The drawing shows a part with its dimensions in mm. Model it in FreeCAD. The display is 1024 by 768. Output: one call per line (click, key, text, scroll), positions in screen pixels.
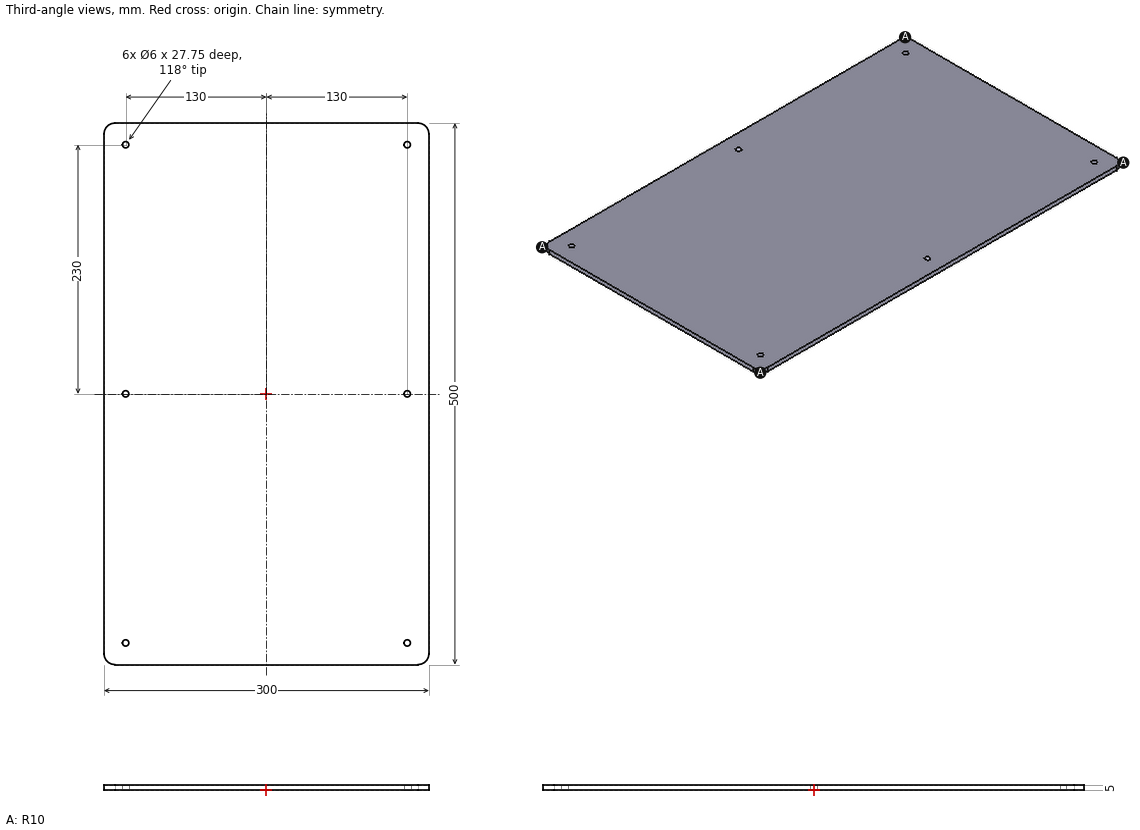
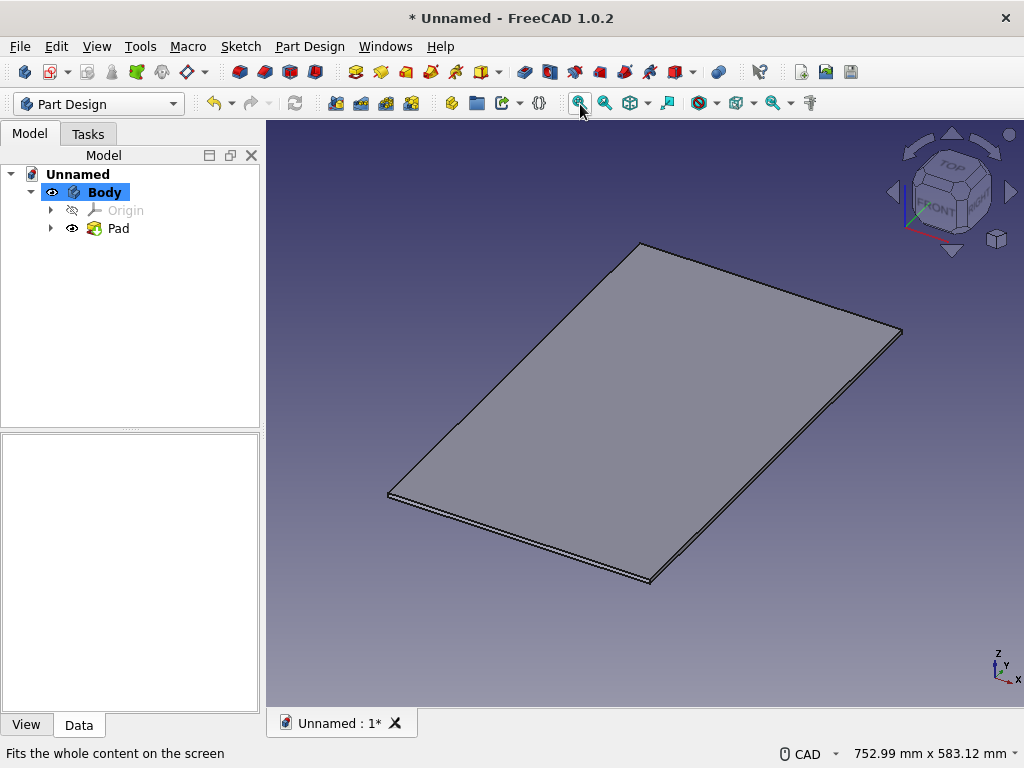
click(681, 375)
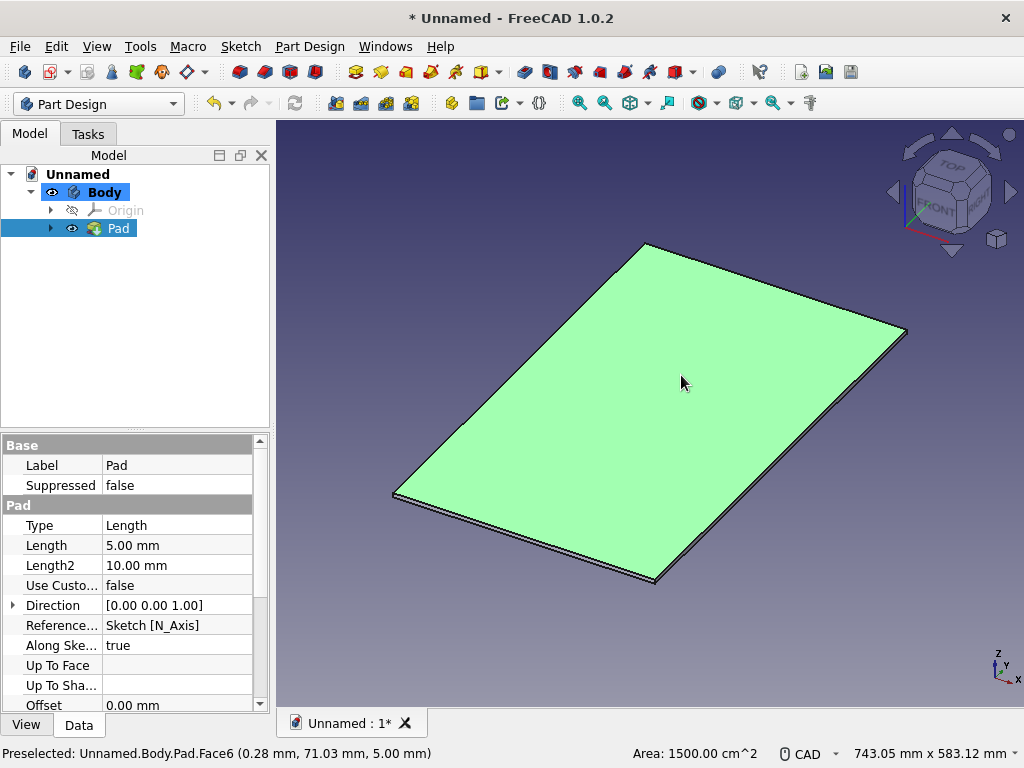
click(50, 72)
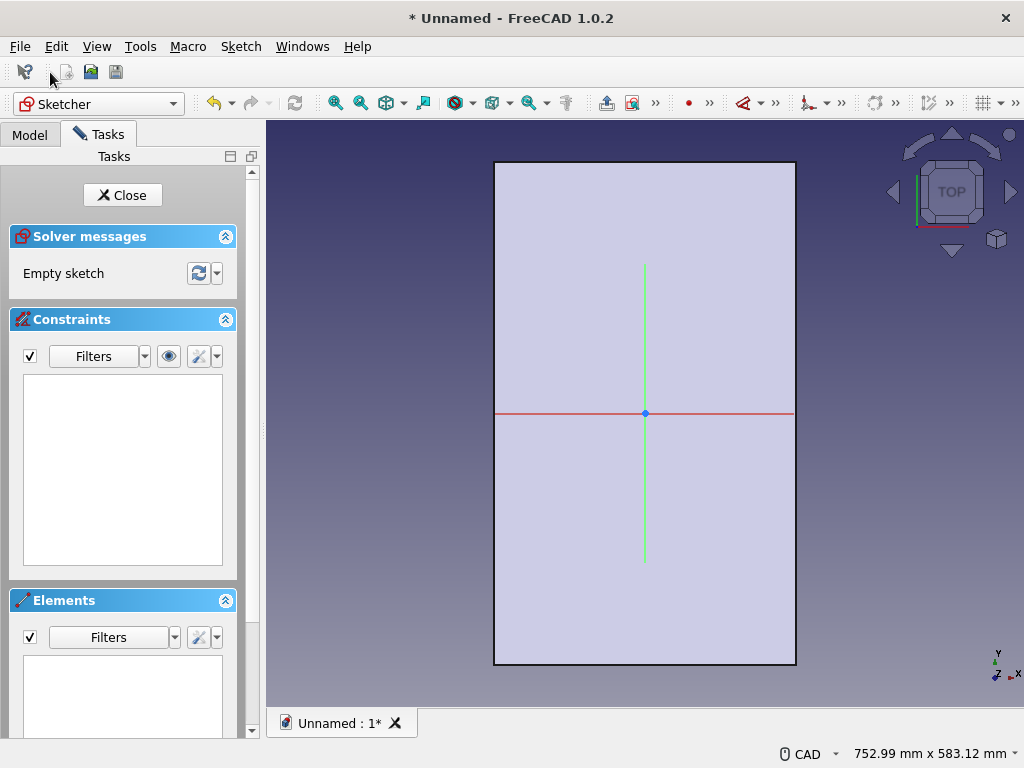
key(g)
key(c)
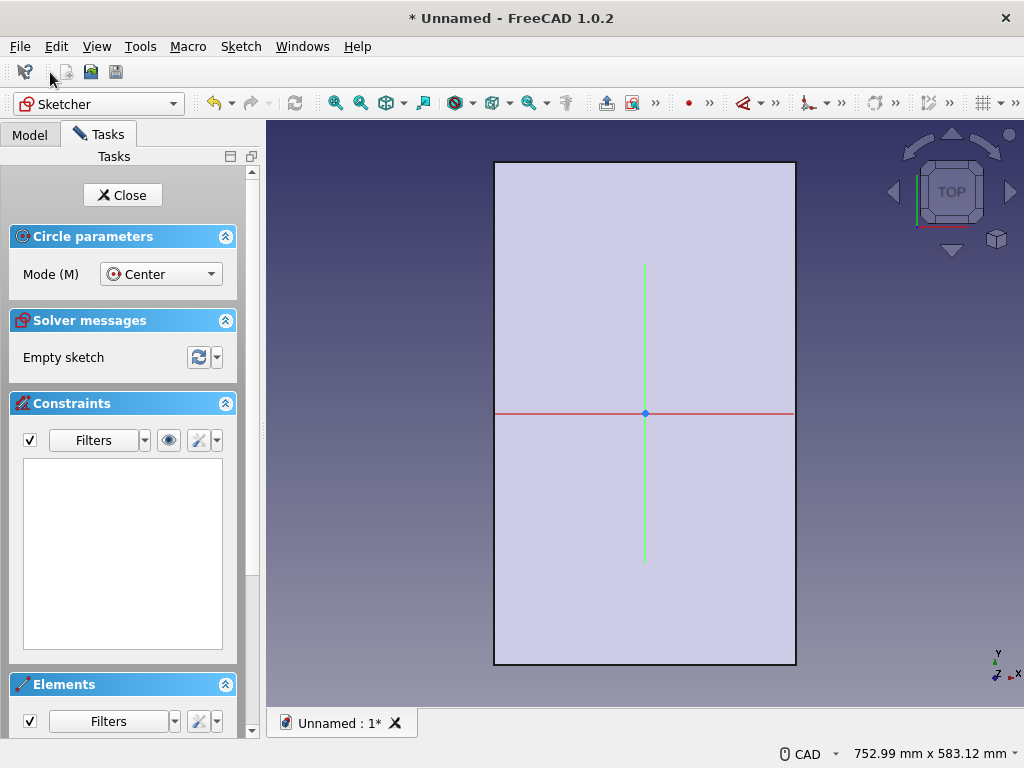
scroll(514, 182, up, 11)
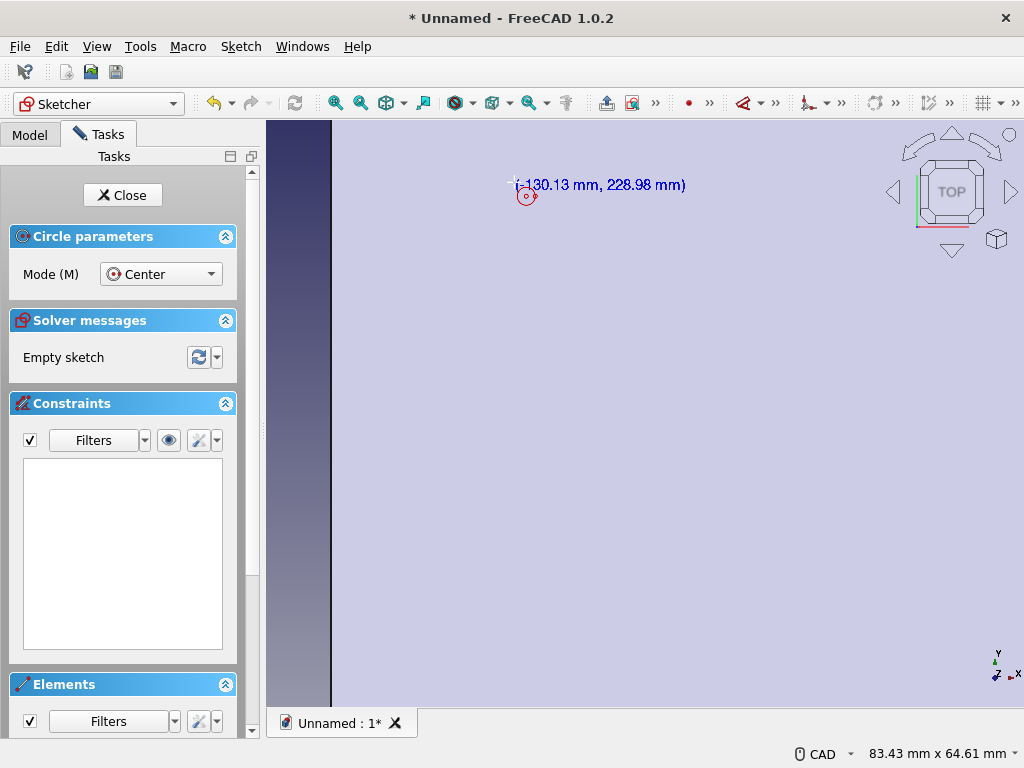
scroll(465, 228, down, 12)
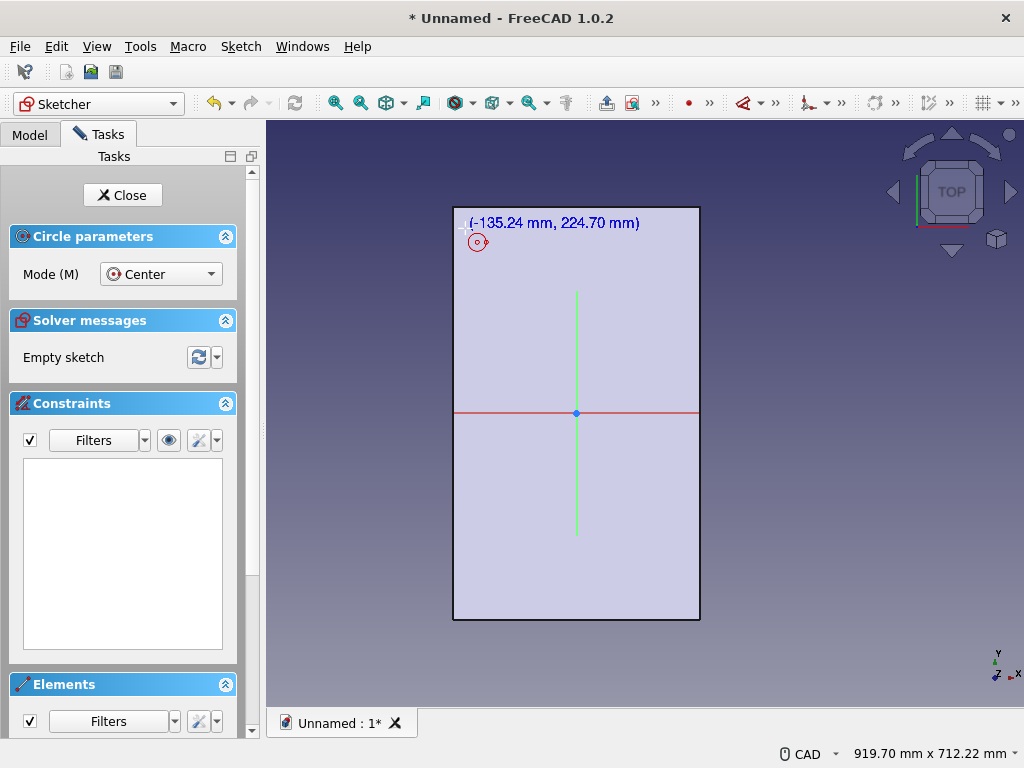
click(470, 224)
move(471, 222)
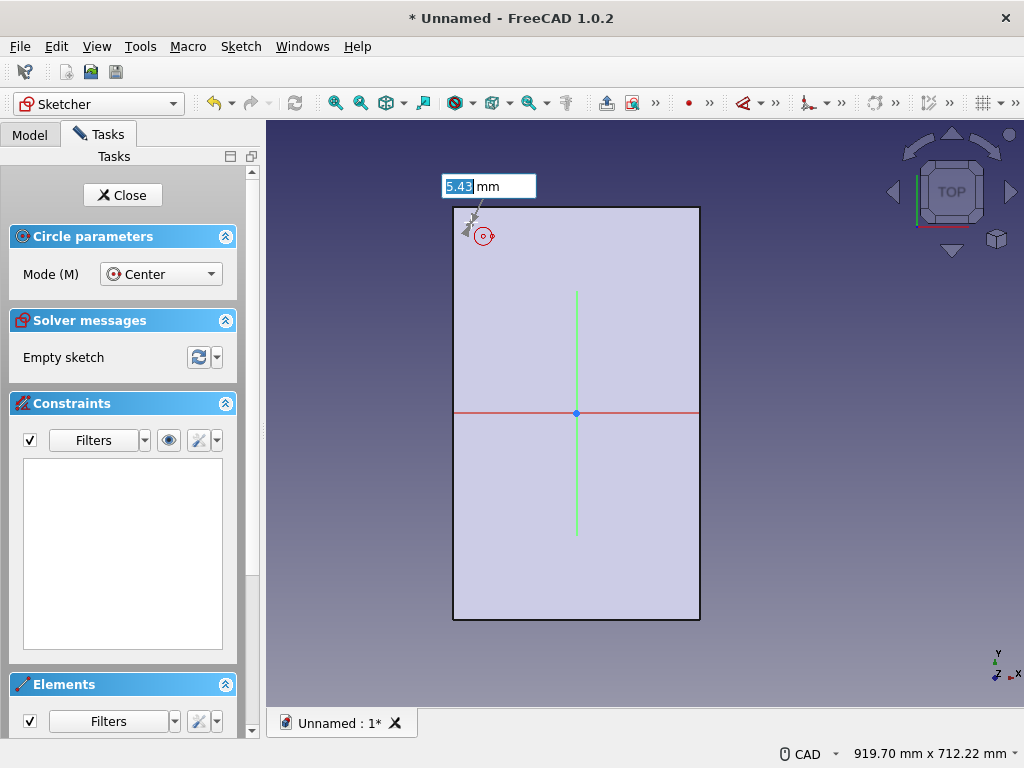
text(6)
key(Return)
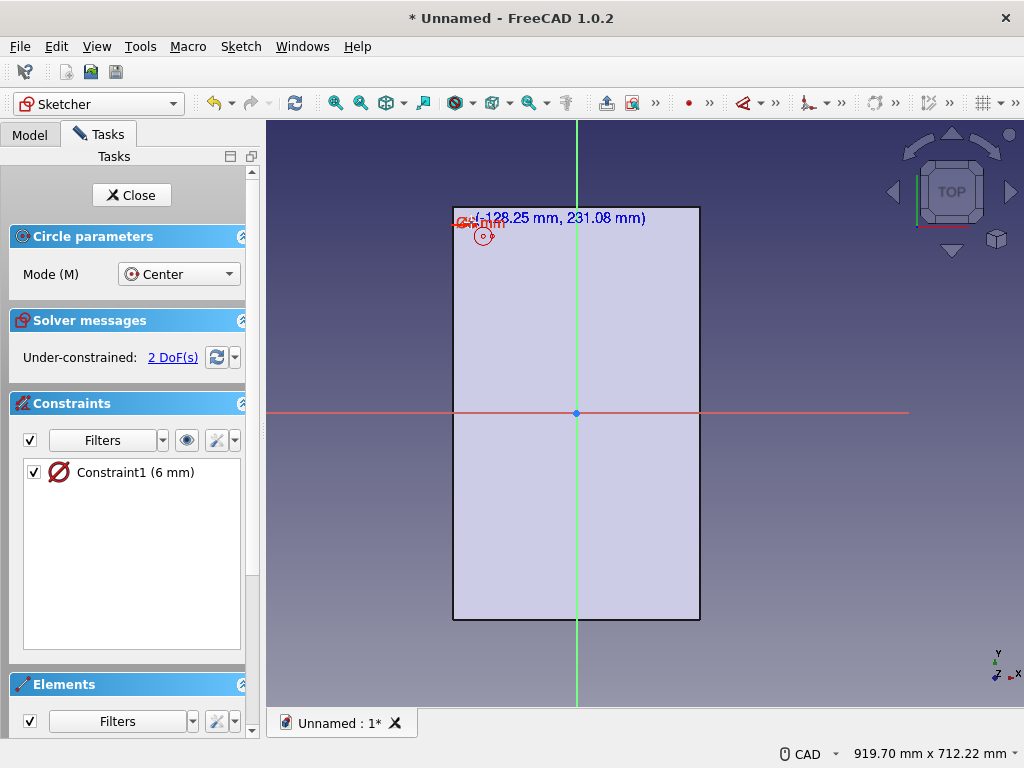
scroll(684, 224, up, 12)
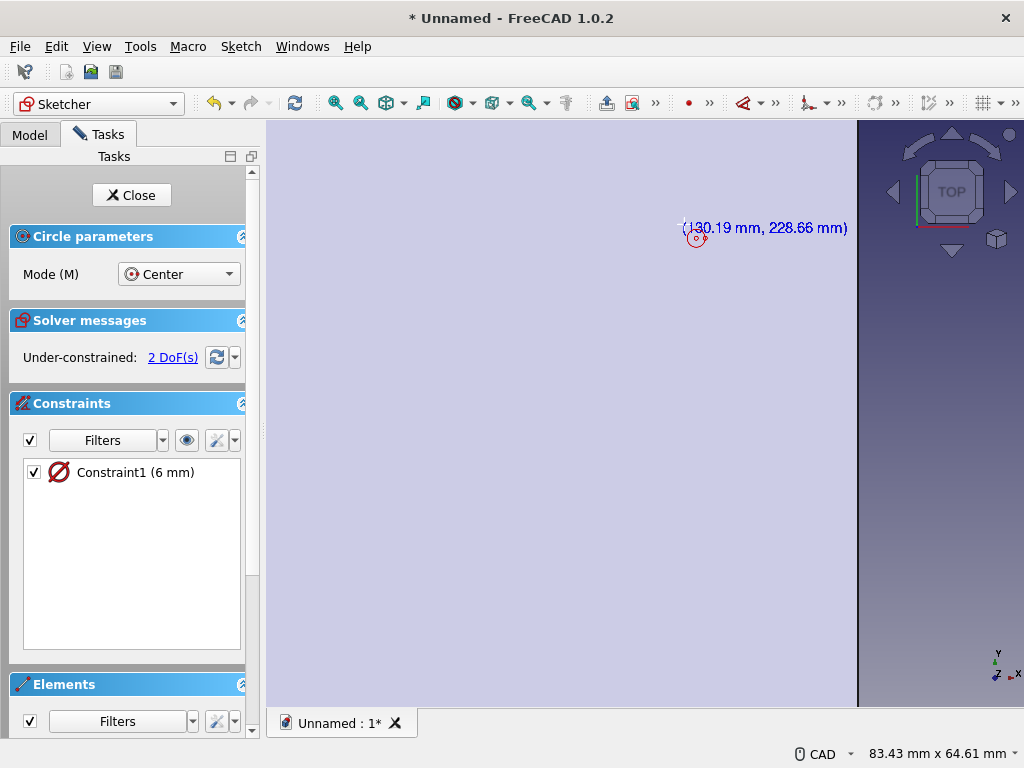
scroll(684, 224, down, 12)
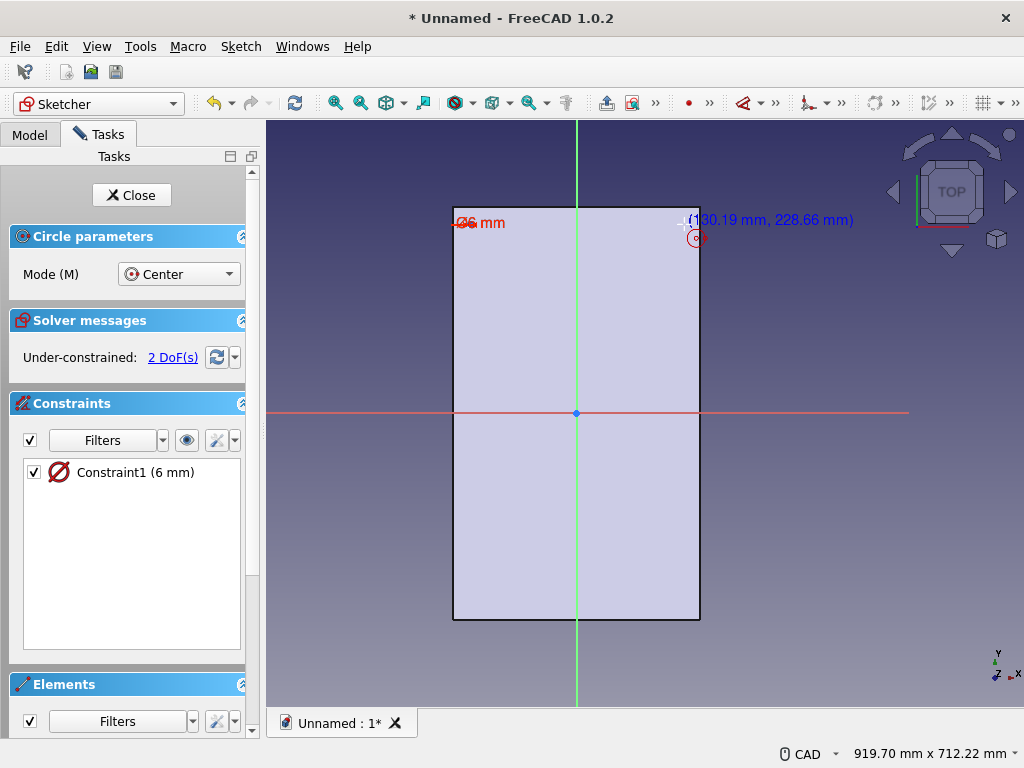
click(684, 224)
move(686, 222)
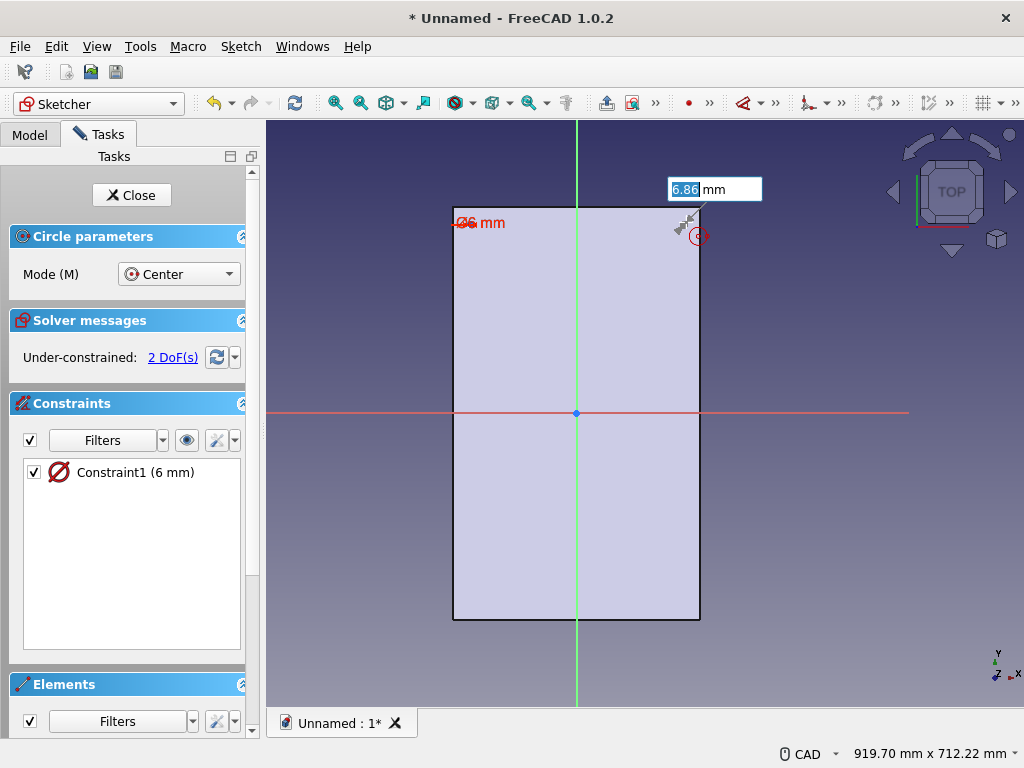
text(6)
key(Return)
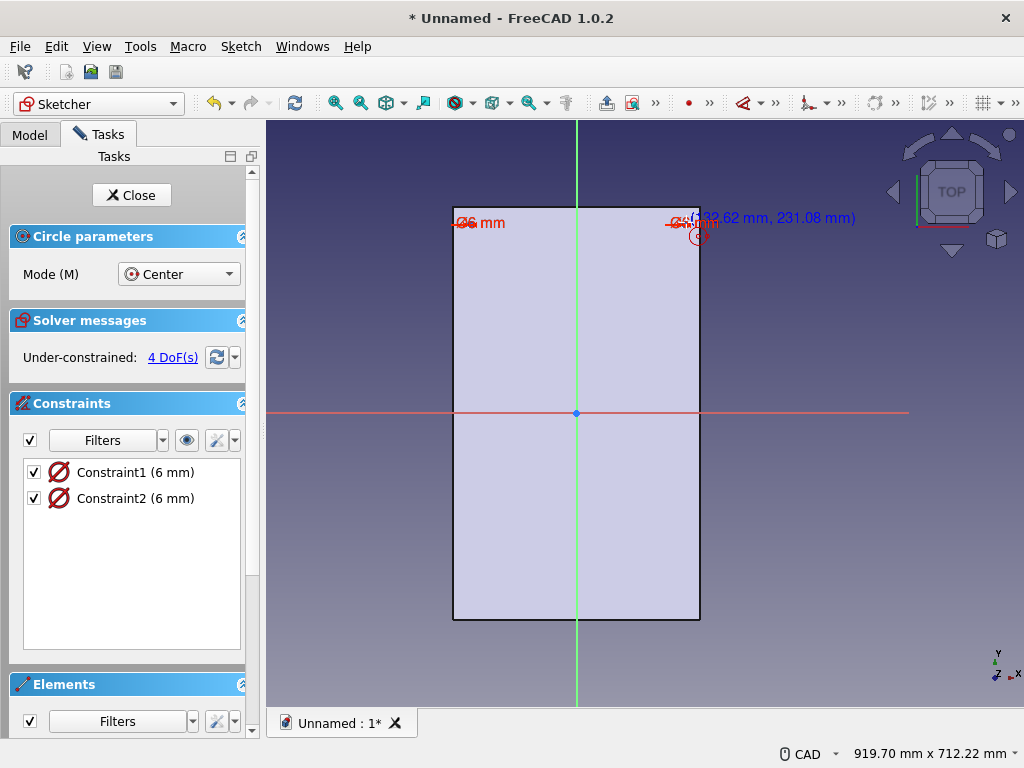
scroll(684, 603, up, 12)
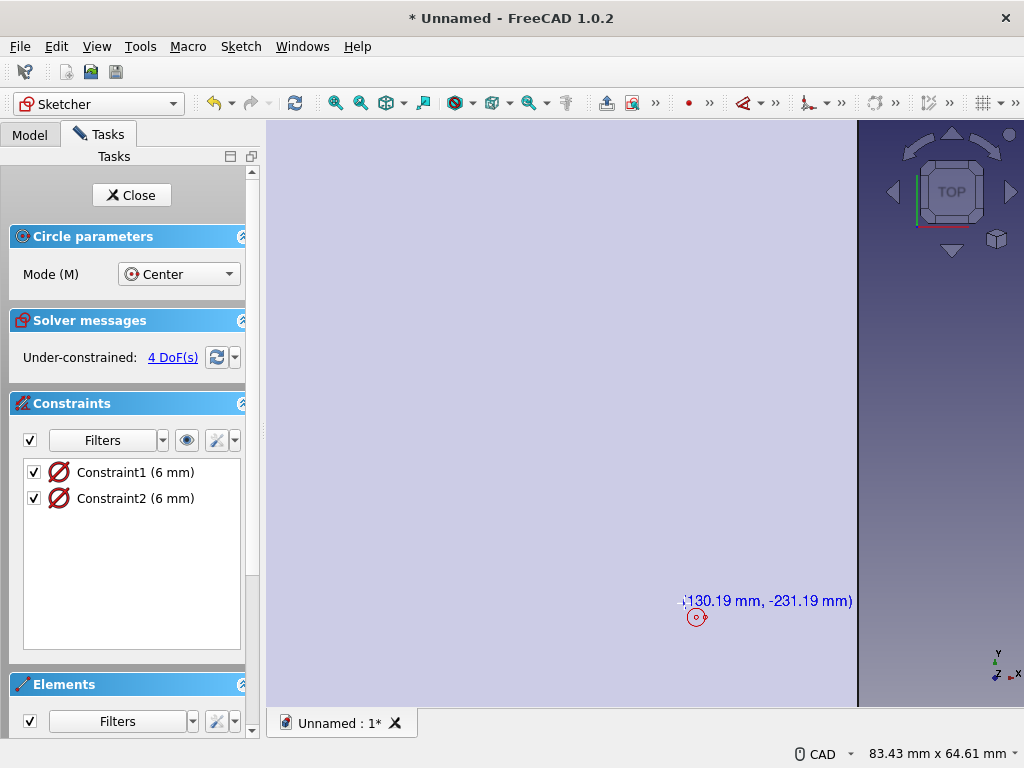
scroll(684, 604, down, 12)